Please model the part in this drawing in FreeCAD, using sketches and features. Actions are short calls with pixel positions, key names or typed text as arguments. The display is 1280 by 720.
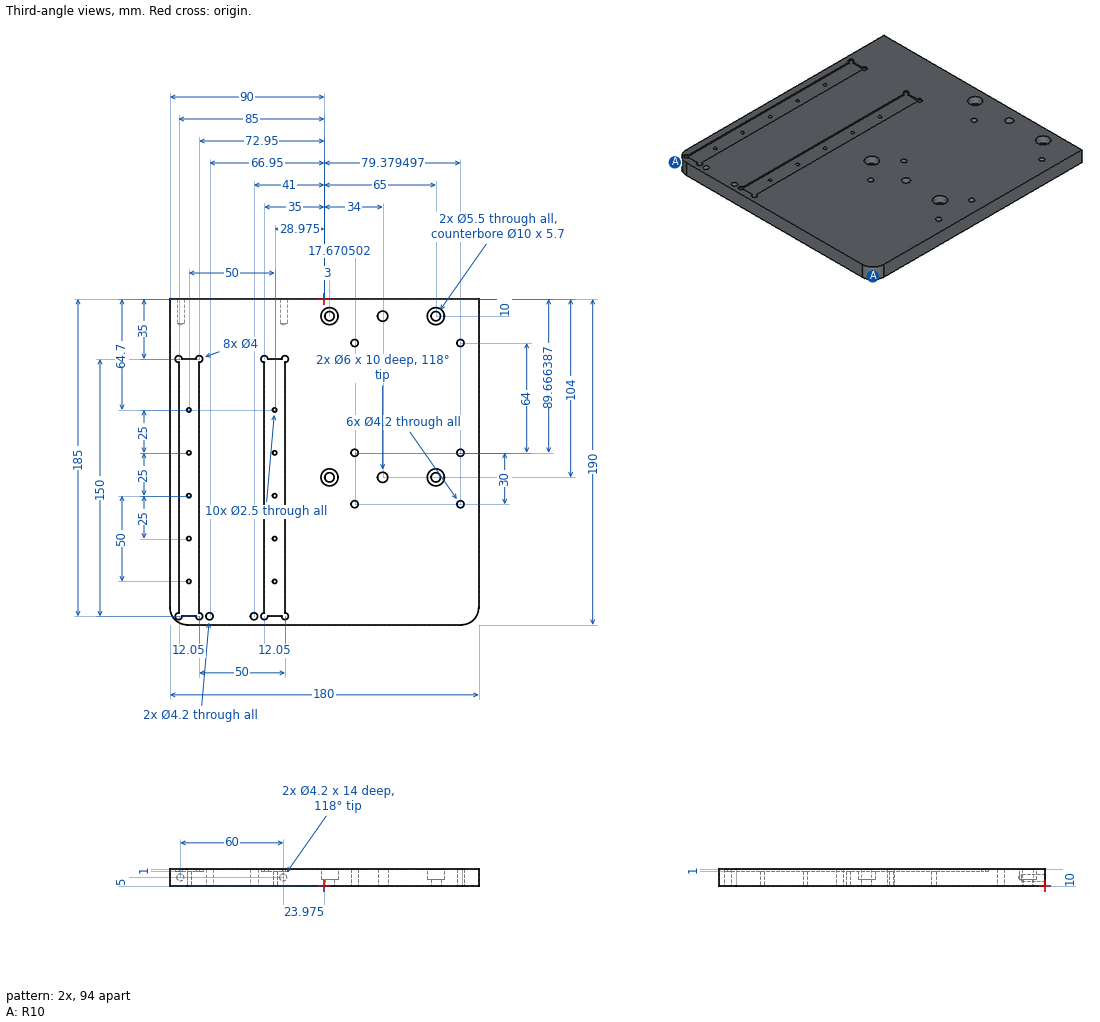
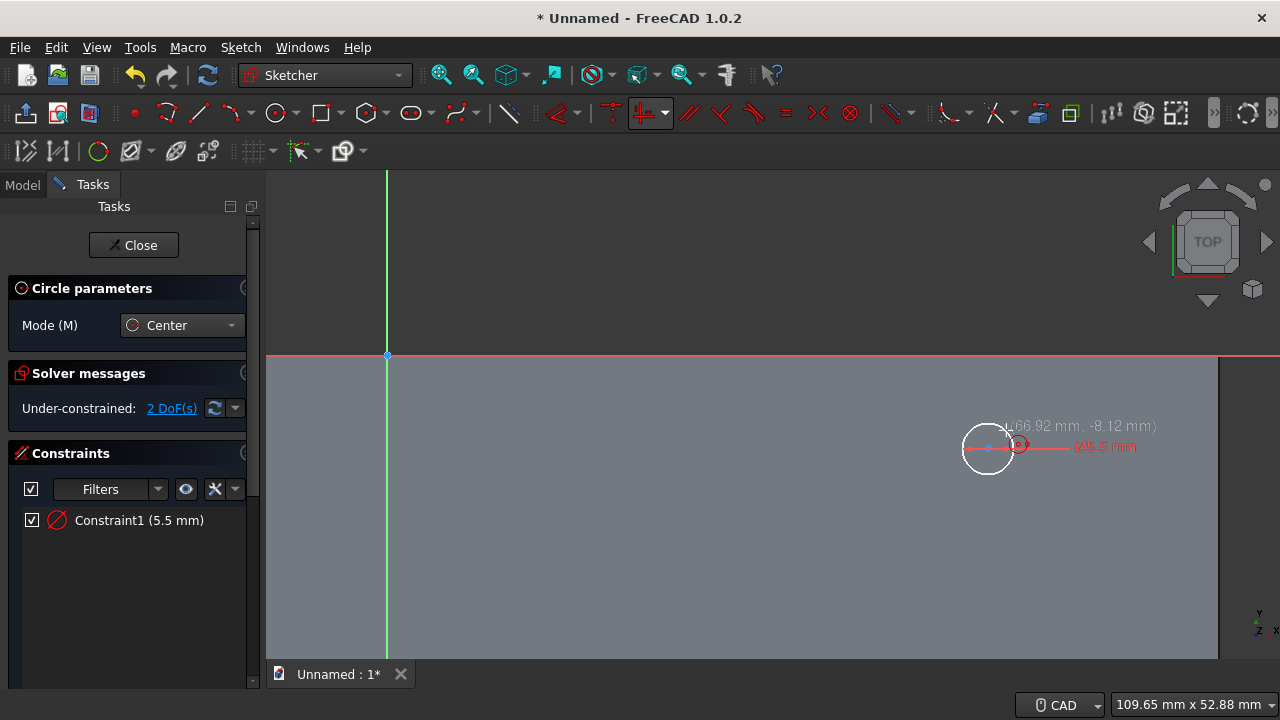
click(415, 448)
move(433, 430)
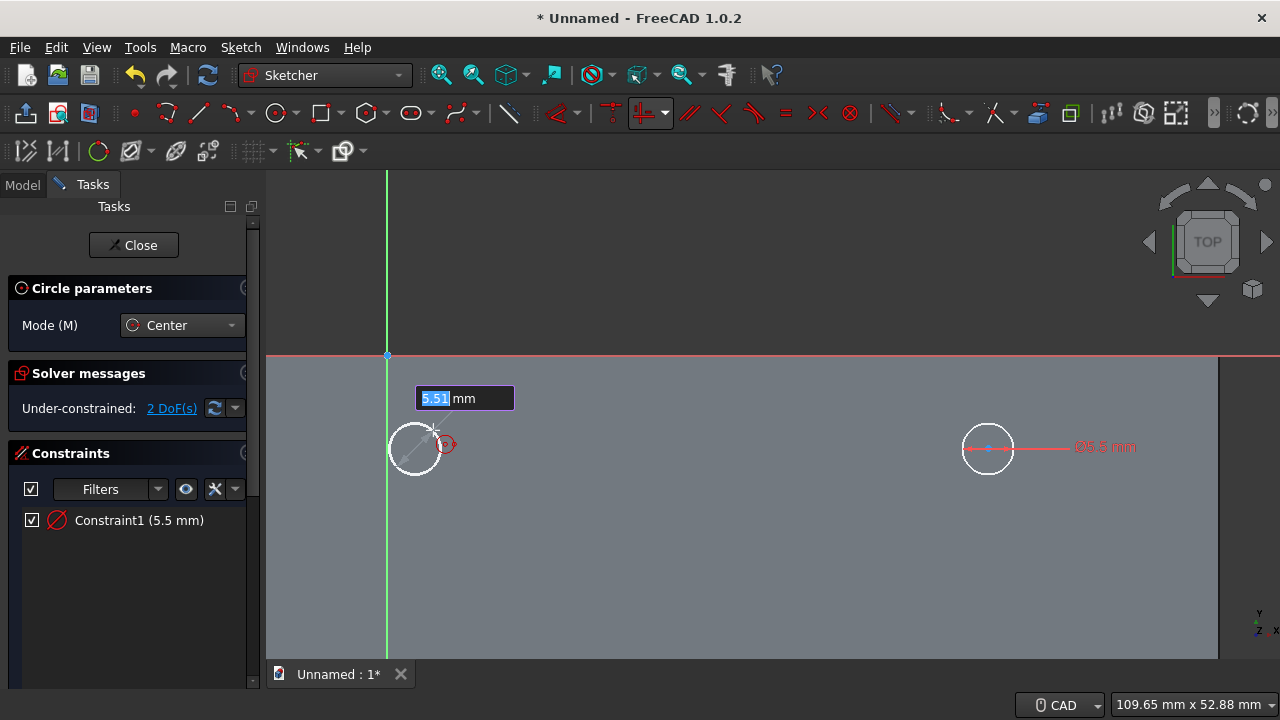
text(5.5)
key(Return)
key(Escape)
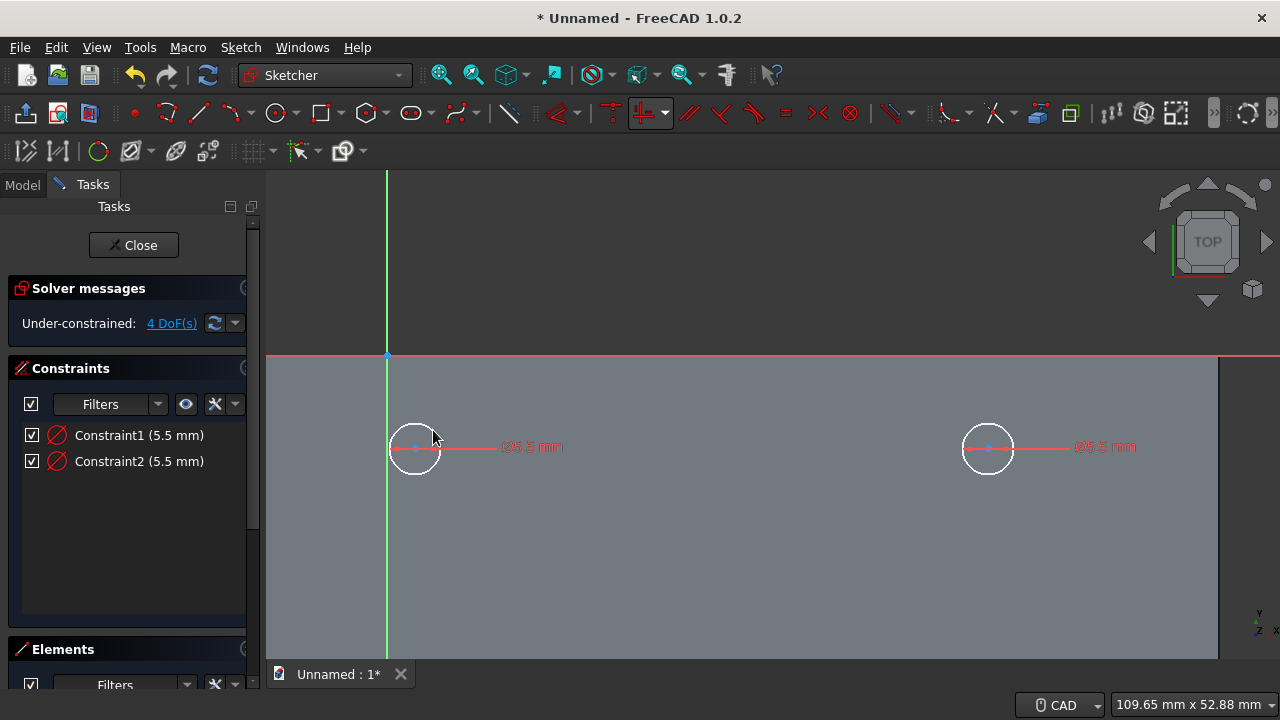
click(988, 449)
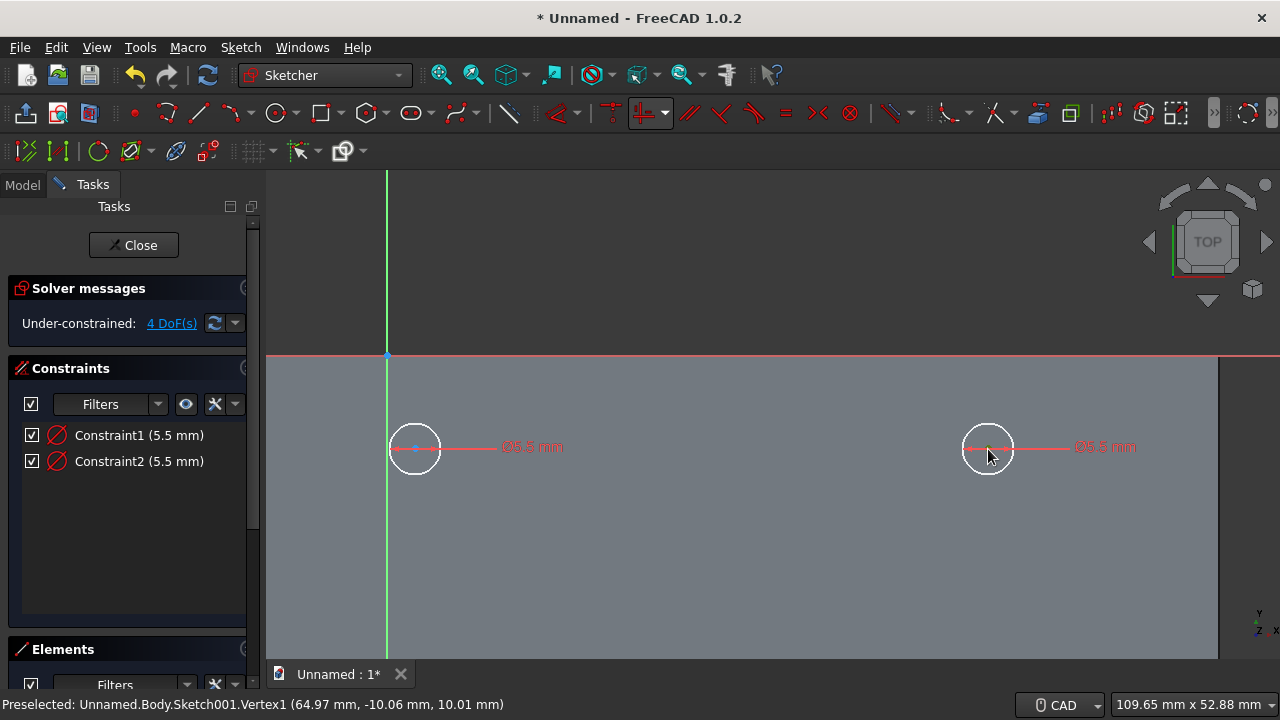
click(415, 449)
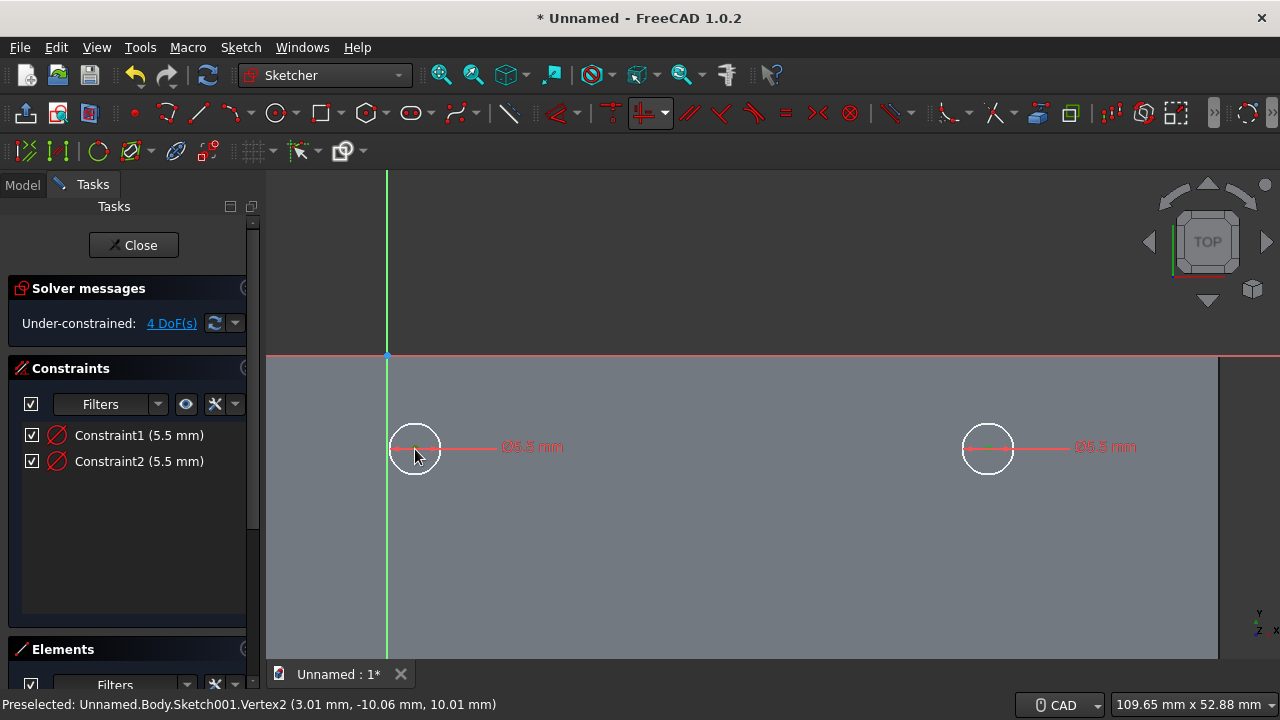
click(668, 114)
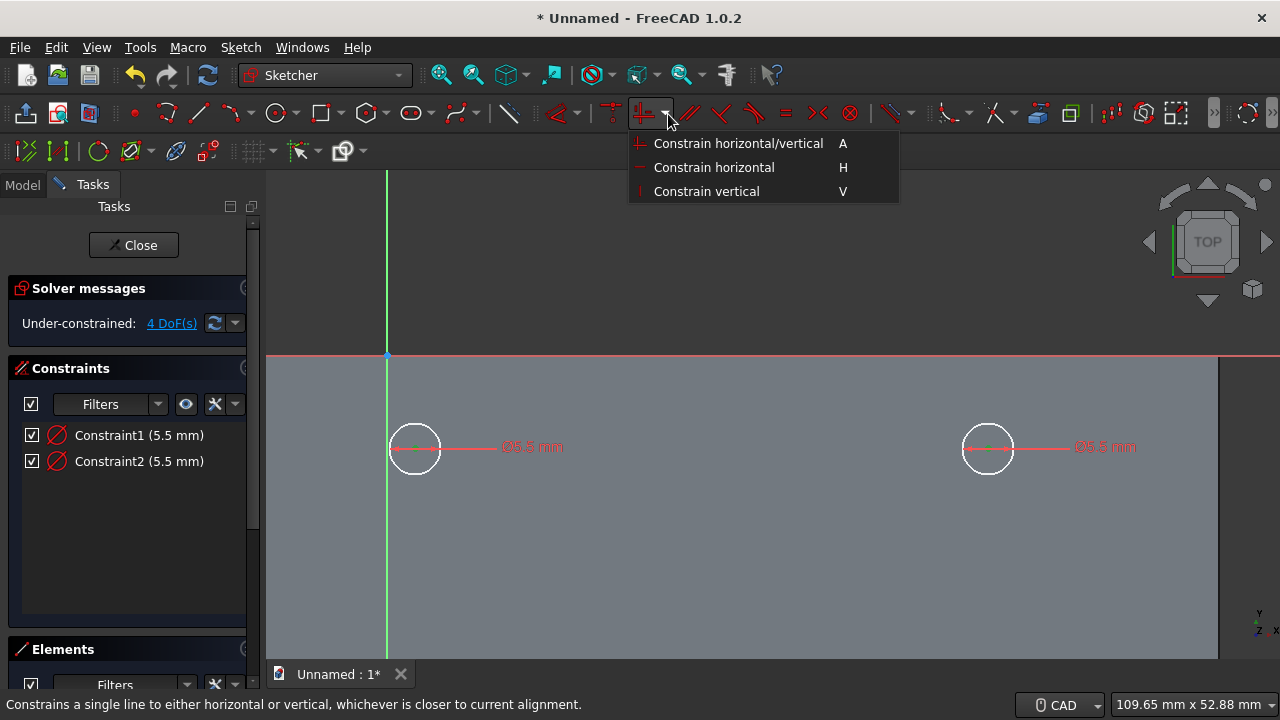
click(764, 167)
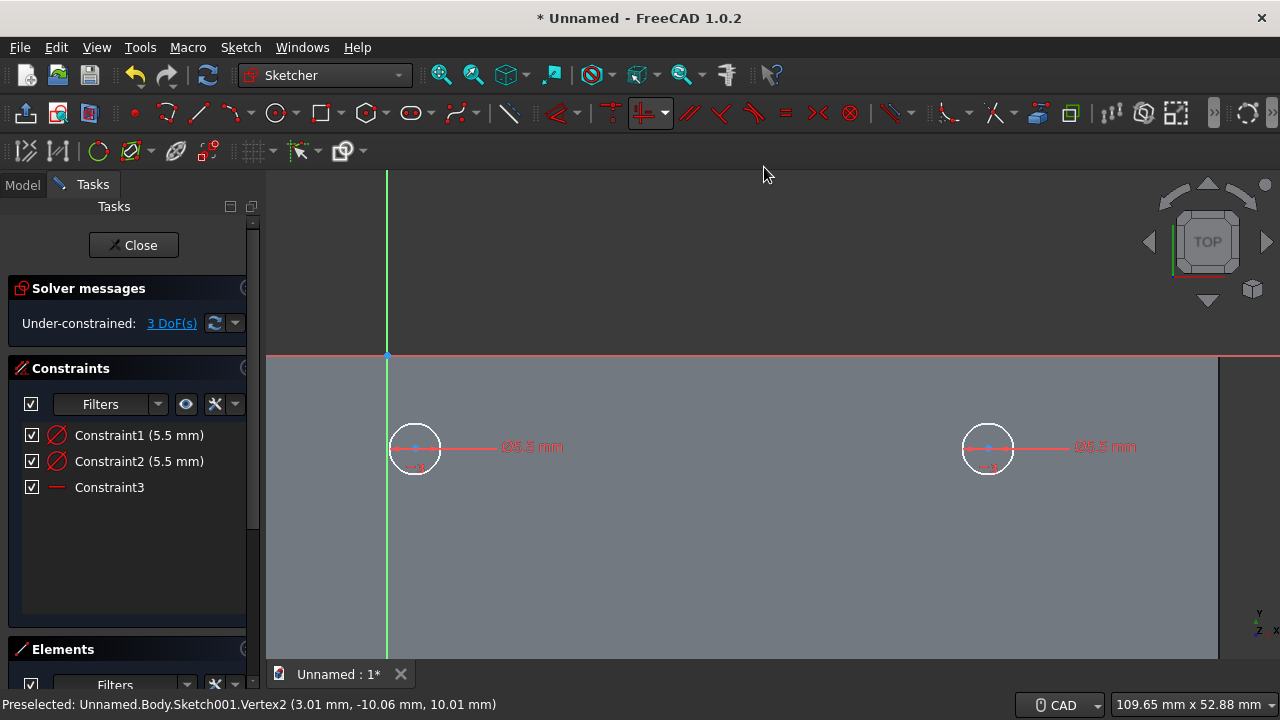
scroll(415, 449, up, 2)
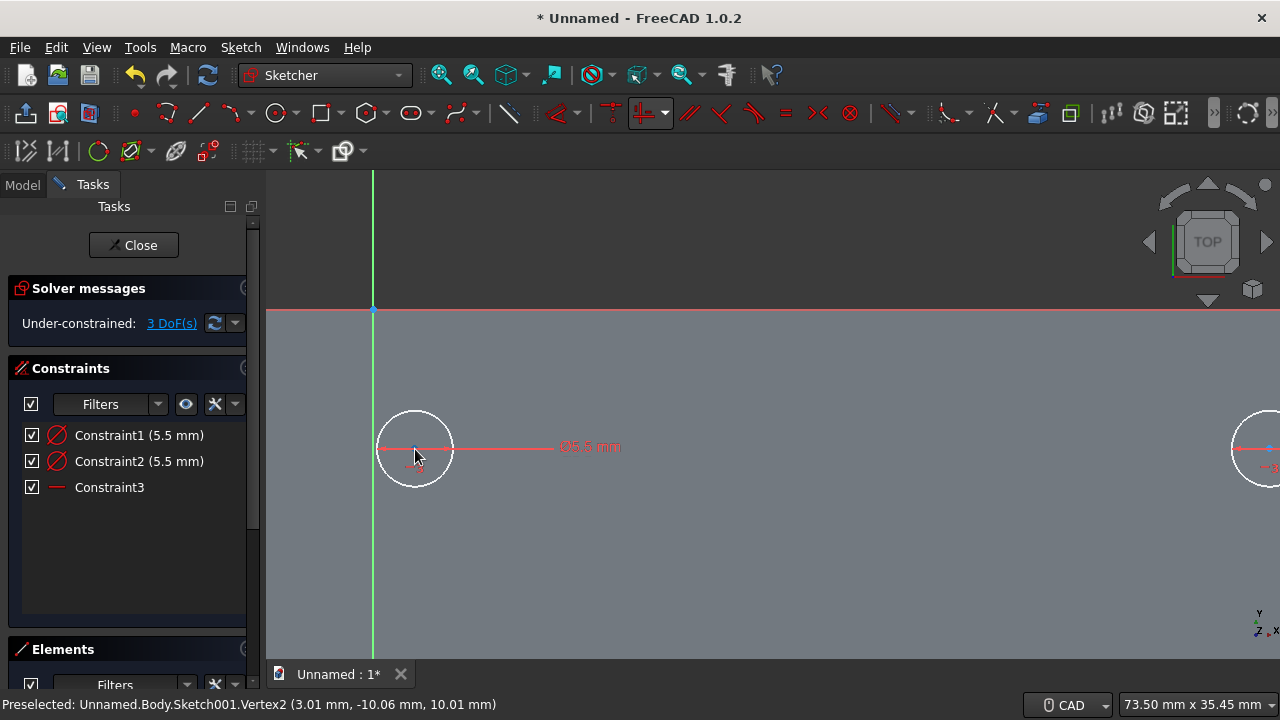
click(415, 449)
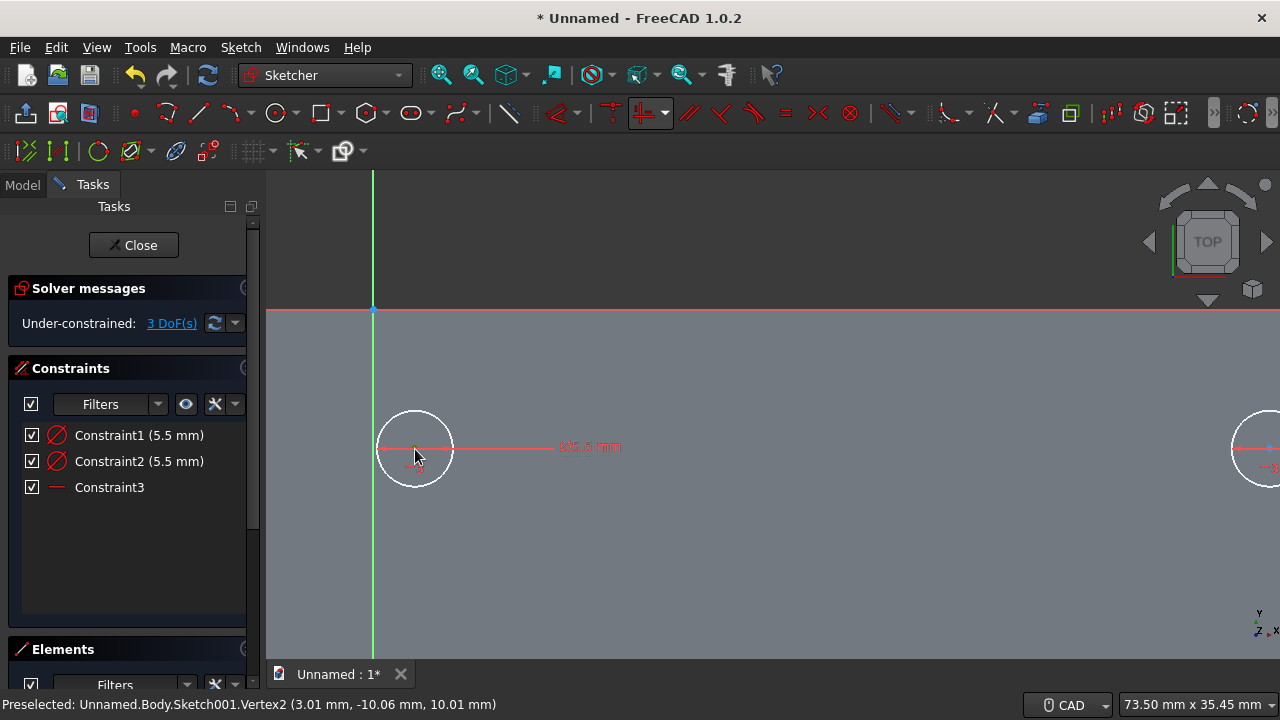
key(l)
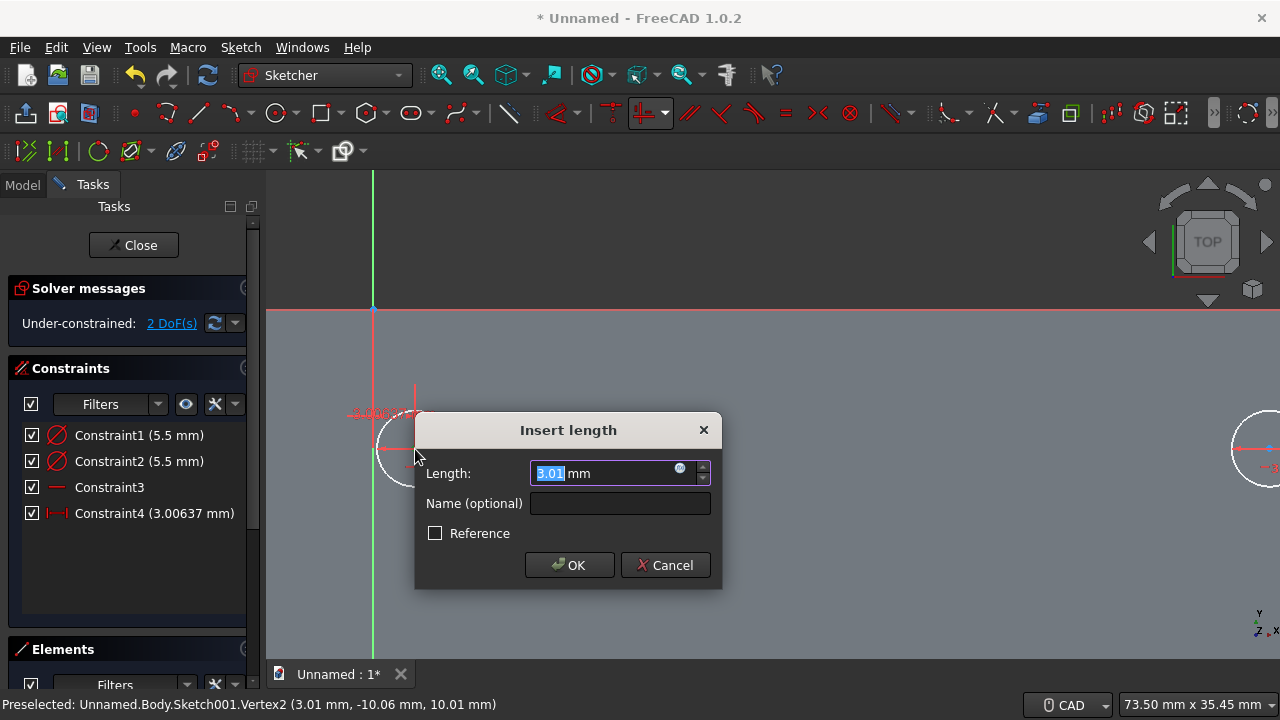
text(3)
key(Return)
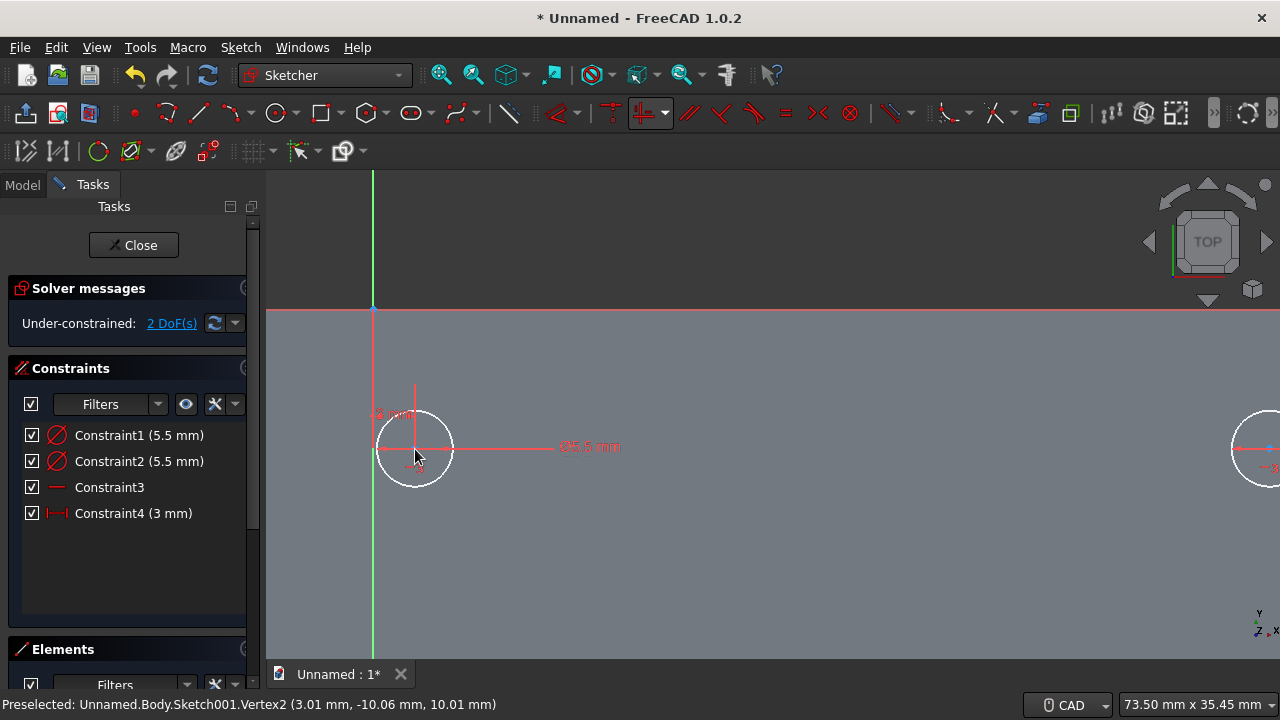
scroll(427, 448, down, 2)